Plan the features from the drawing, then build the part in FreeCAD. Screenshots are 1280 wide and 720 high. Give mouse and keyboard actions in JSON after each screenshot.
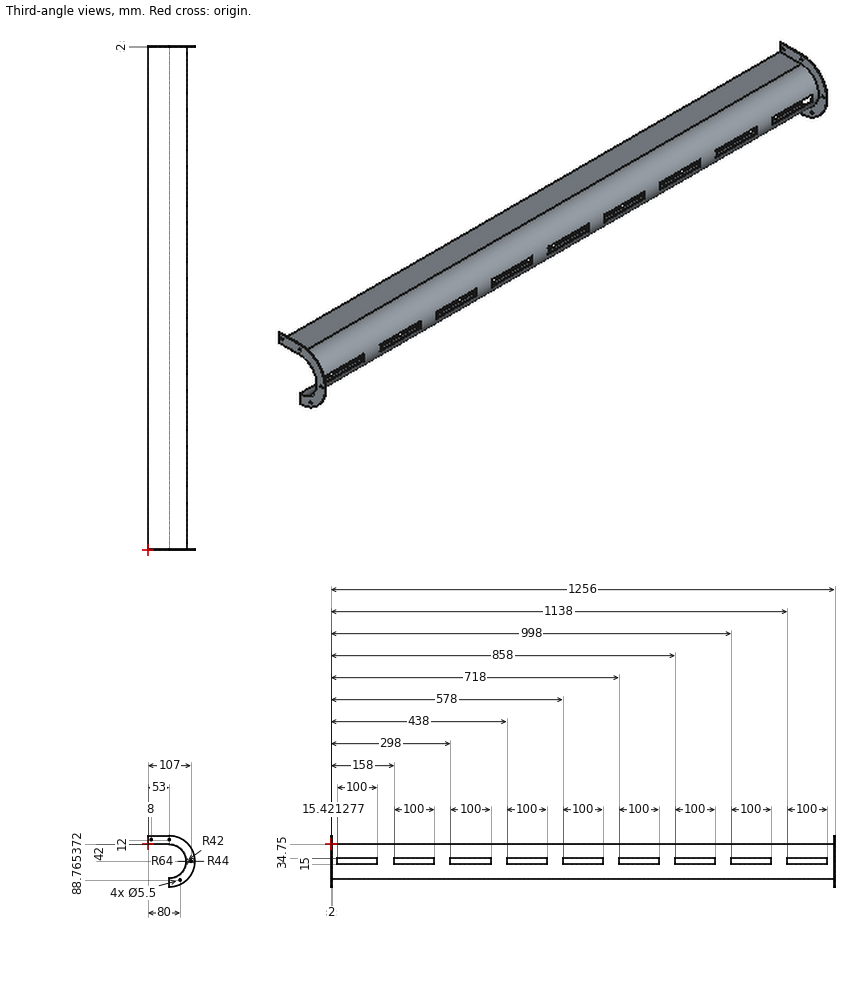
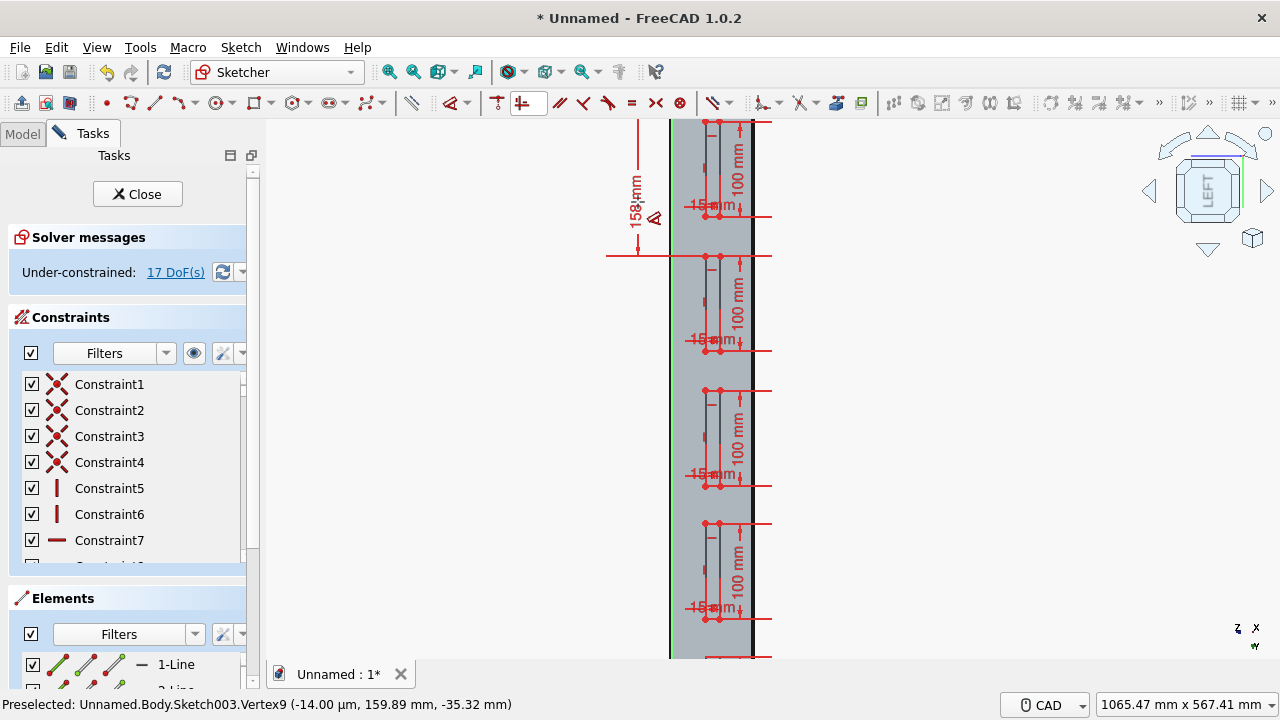
{"action": "scroll", "coordinate": [708, 257], "scroll_direction": "down", "scroll_amount": 6}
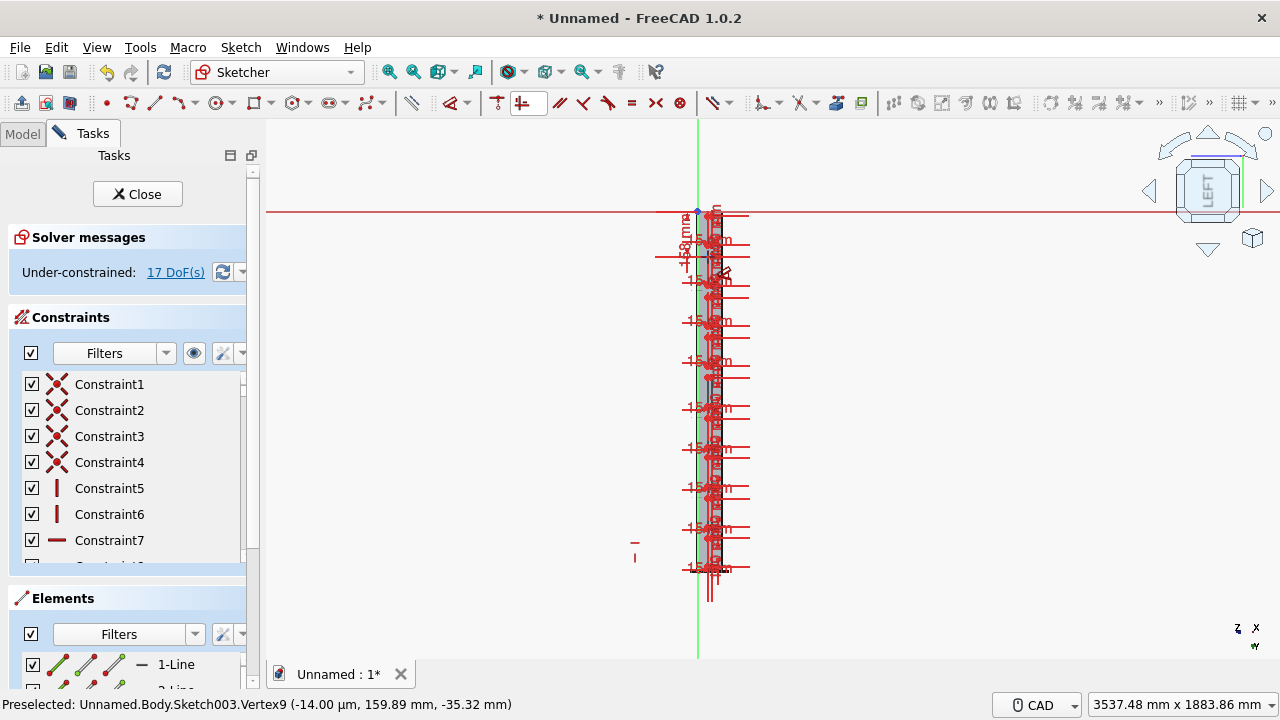
{"action": "scroll", "coordinate": [708, 499], "scroll_direction": "up", "scroll_amount": 6}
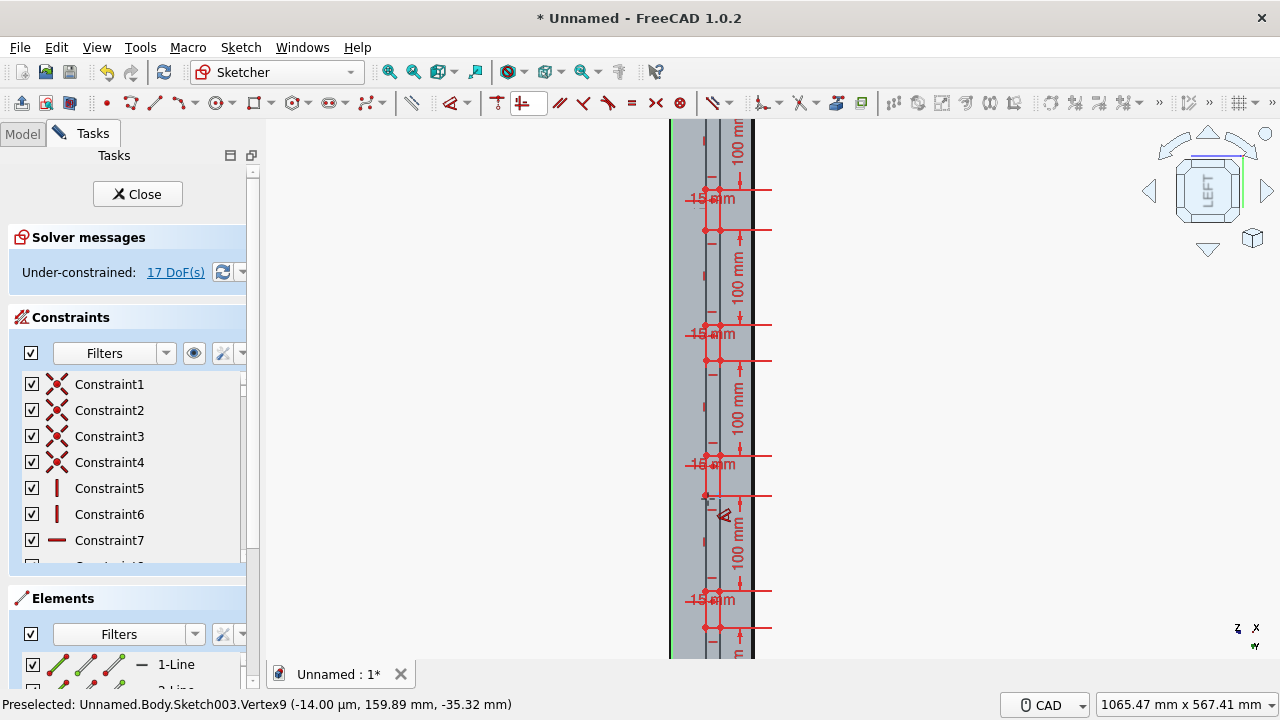
{"action": "left_click", "coordinate": [706, 496]}
{"action": "left_click", "coordinate": [638, 321]}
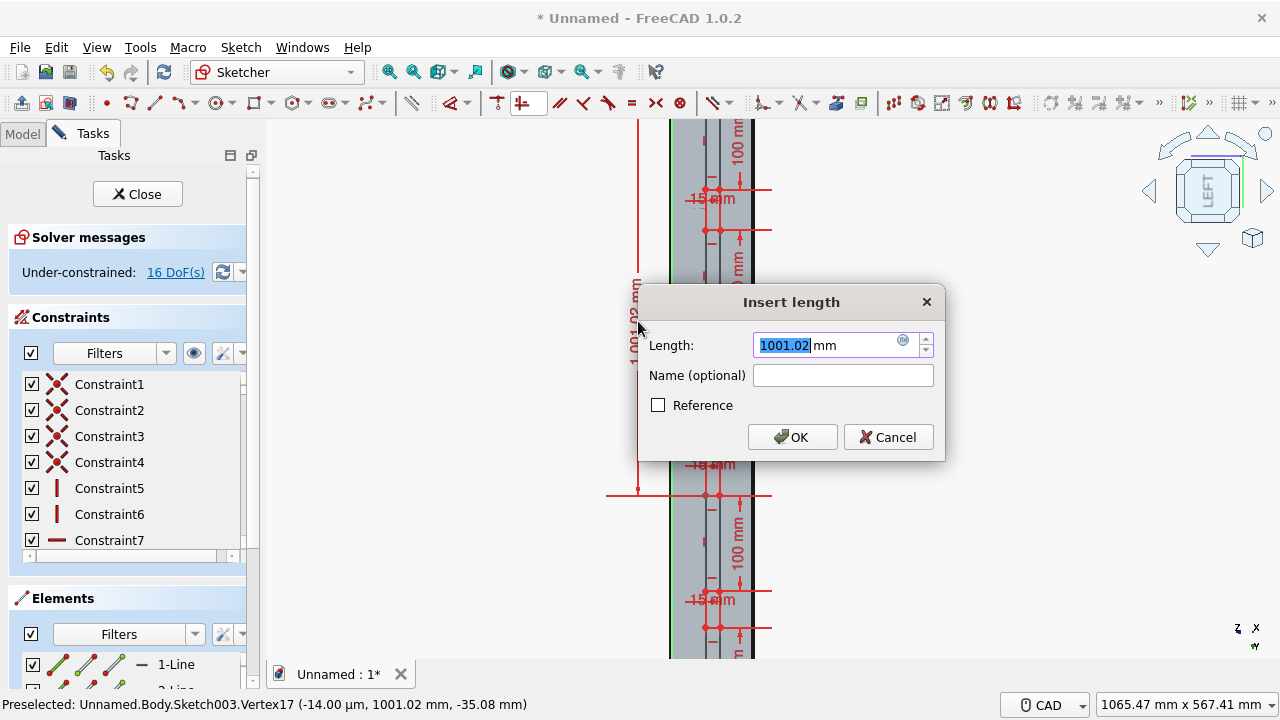
{"action": "type", "text": "998"}
{"action": "key", "text": "Return"}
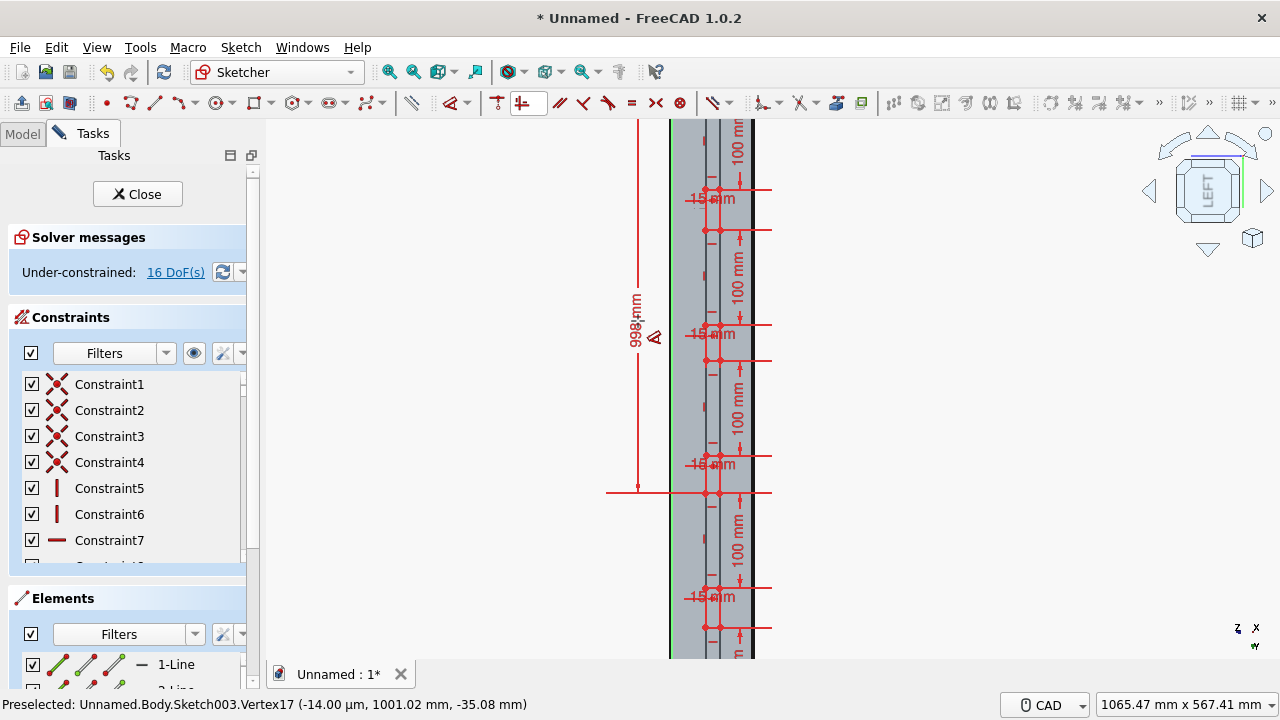
{"action": "scroll", "coordinate": [708, 500], "scroll_direction": "down", "scroll_amount": 6}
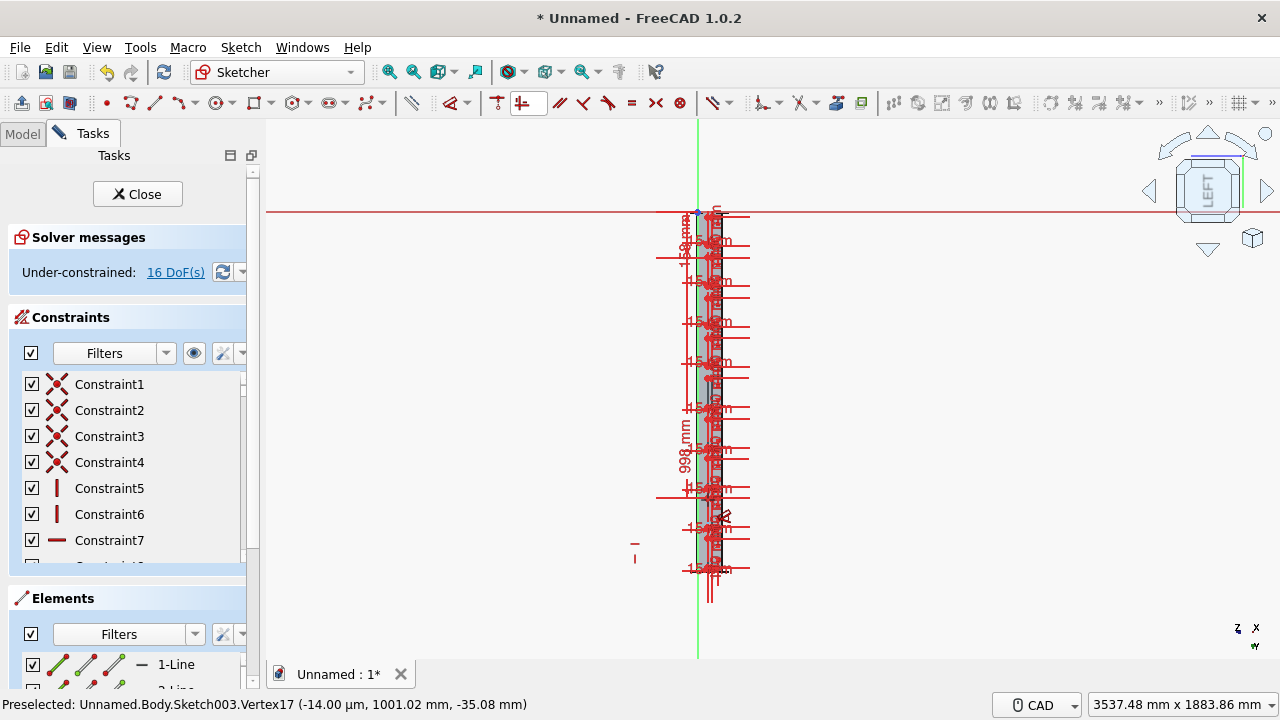
{"action": "scroll", "coordinate": [708, 298], "scroll_direction": "up", "scroll_amount": 6}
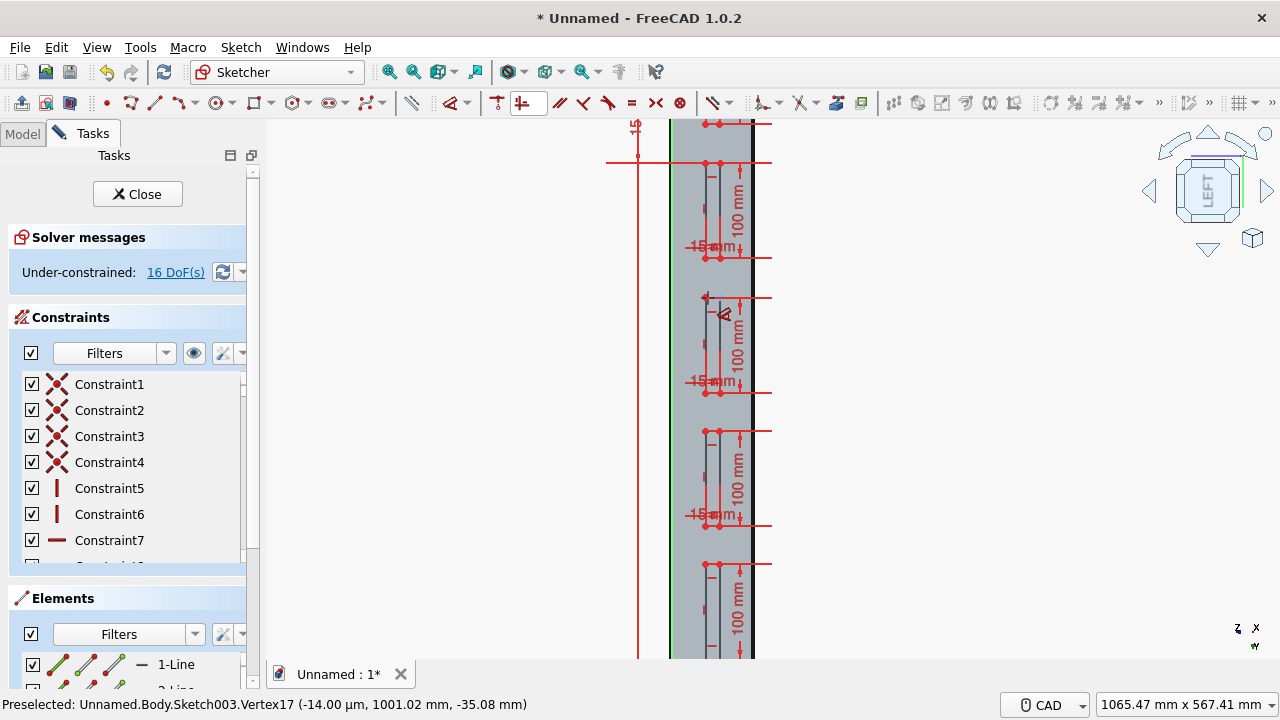
{"action": "left_click", "coordinate": [706, 298]}
{"action": "left_click", "coordinate": [638, 222]}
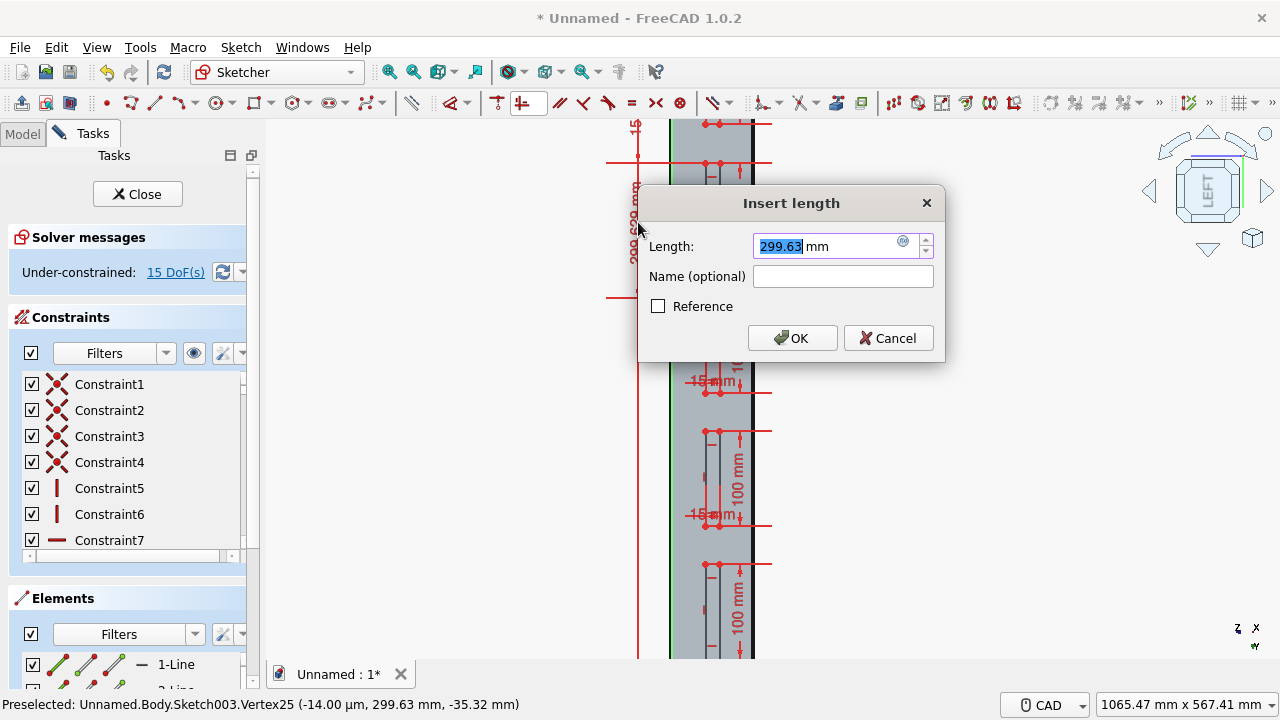
{"action": "type", "text": "298"}
{"action": "key", "text": "Return"}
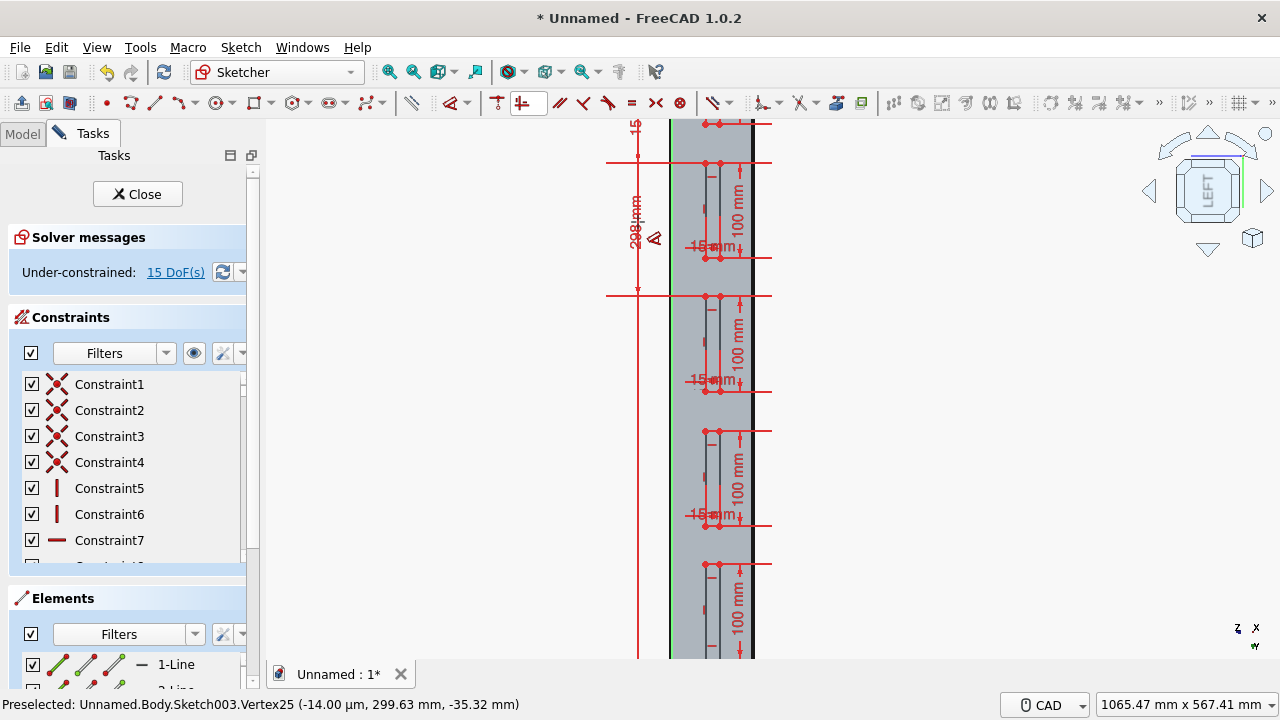
{"action": "left_click", "coordinate": [706, 431]}
{"action": "left_click", "coordinate": [638, 289]}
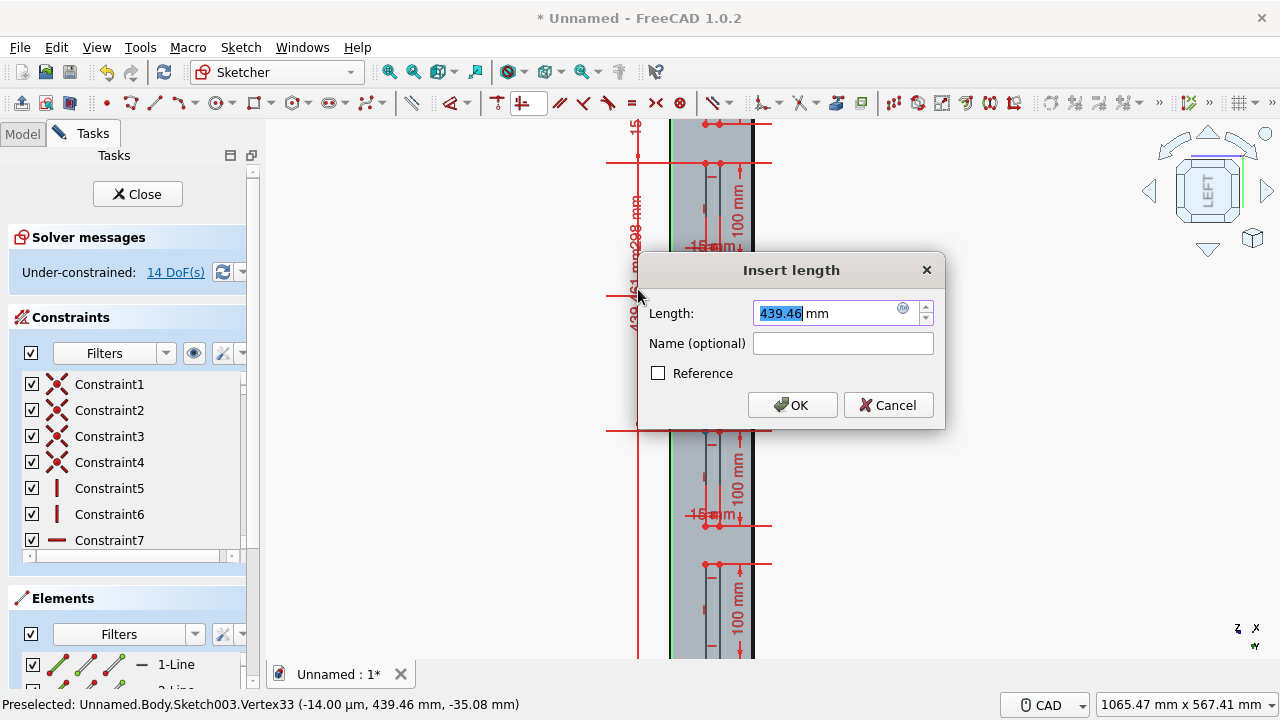
{"action": "type", "text": "438"}
{"action": "key", "text": "Return"}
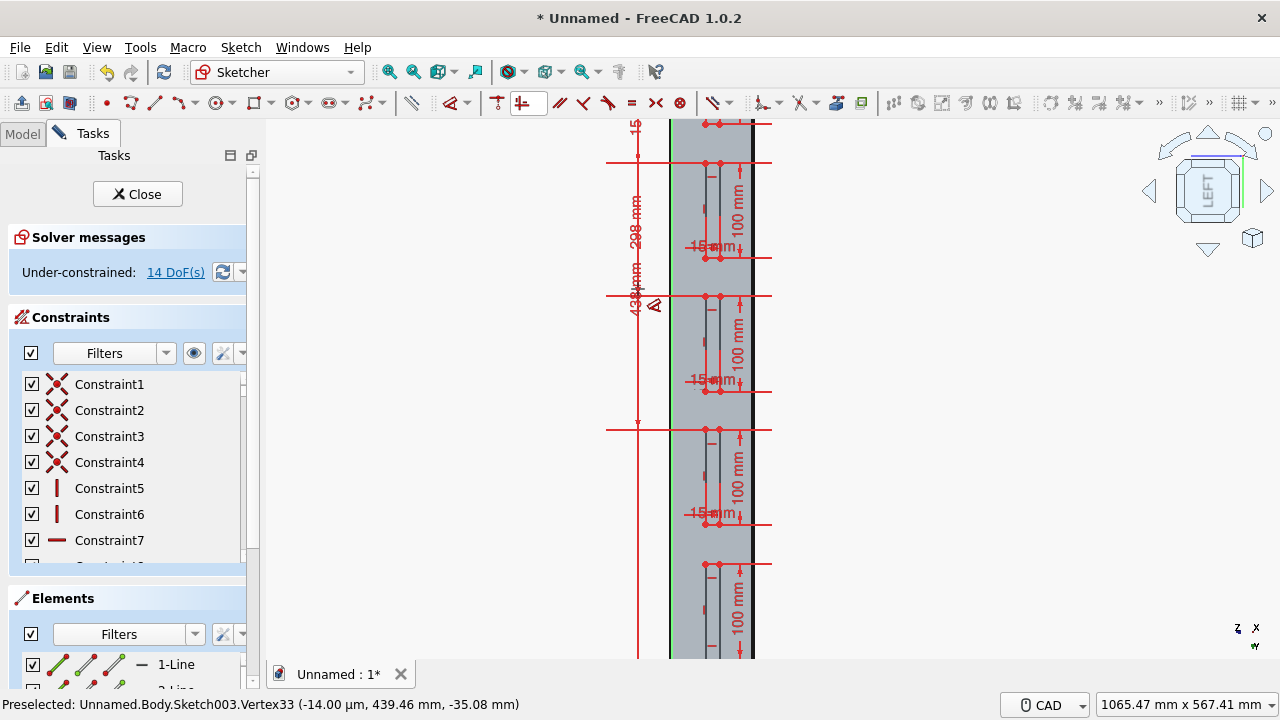
{"action": "left_click", "coordinate": [706, 564]}
{"action": "left_click", "coordinate": [638, 356]}